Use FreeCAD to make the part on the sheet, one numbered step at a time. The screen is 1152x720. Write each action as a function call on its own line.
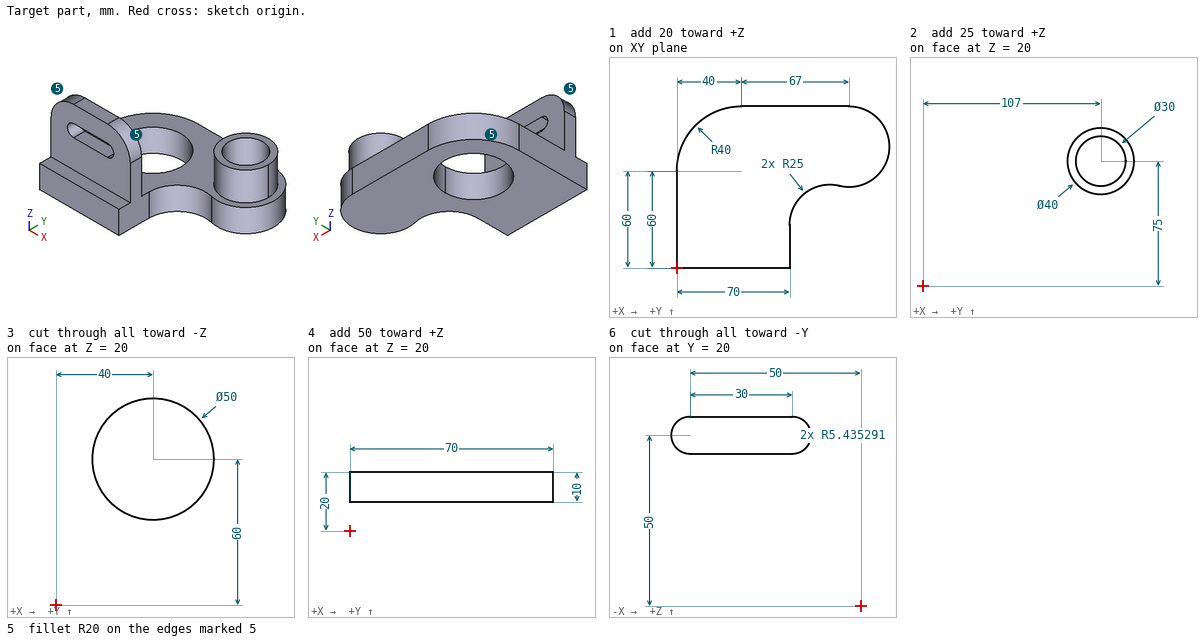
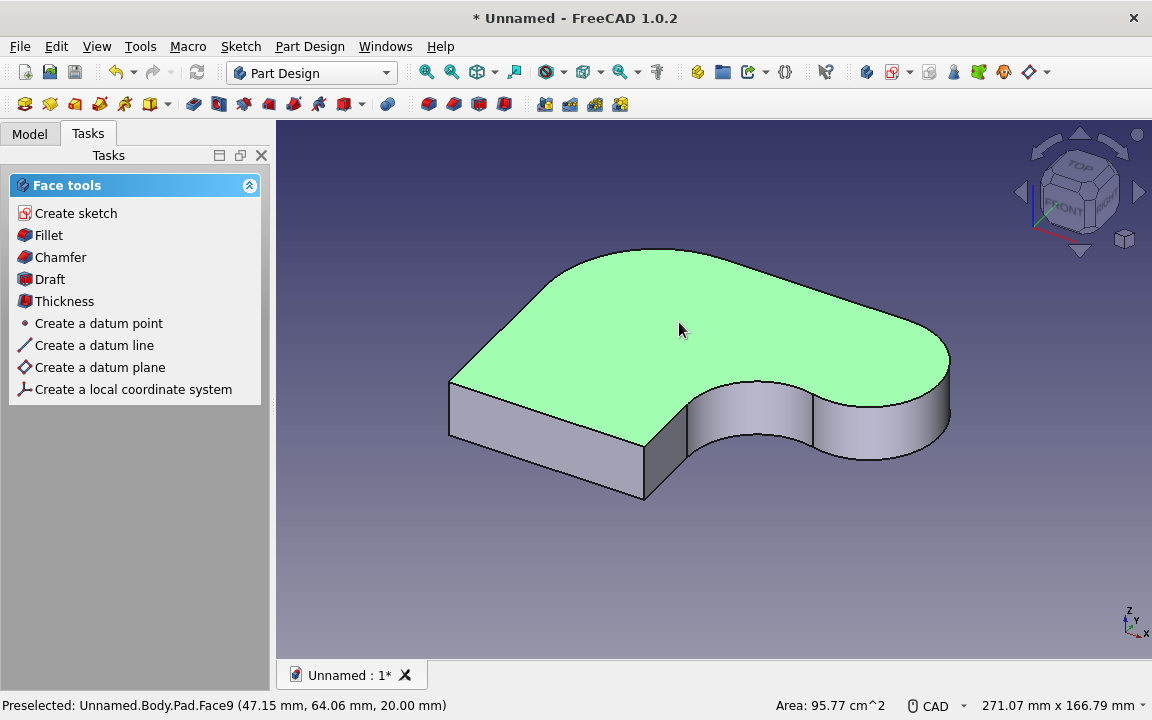
click(892, 72)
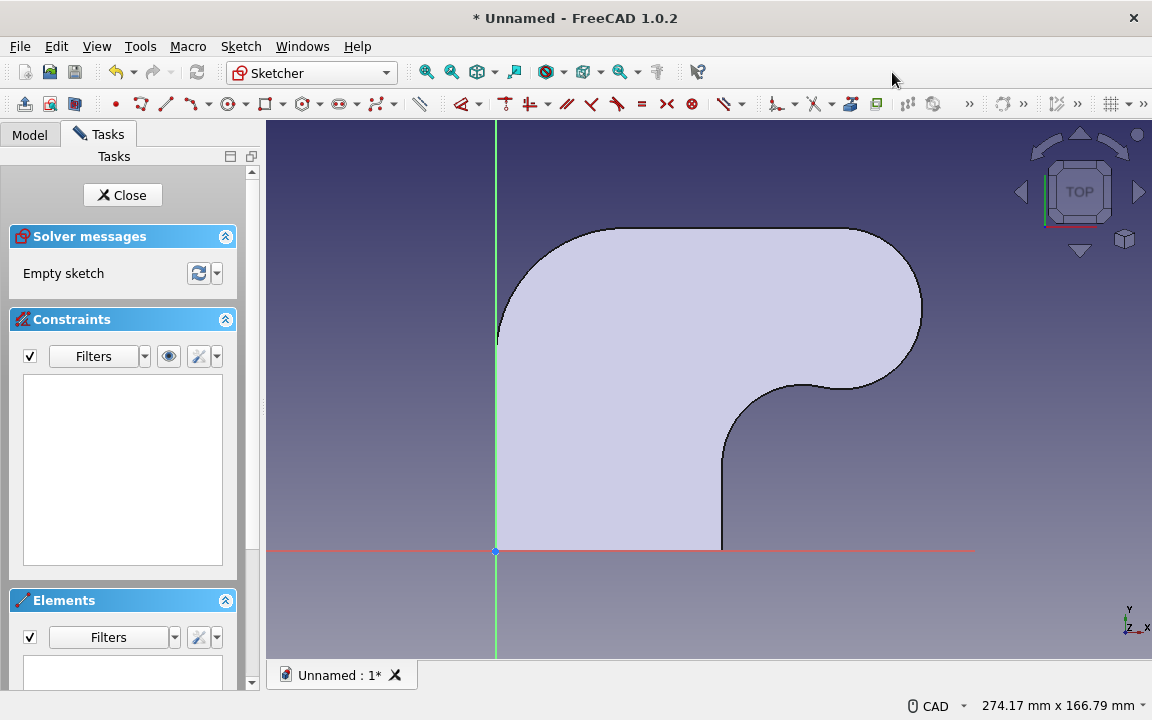
scroll(959, 262, up, 5)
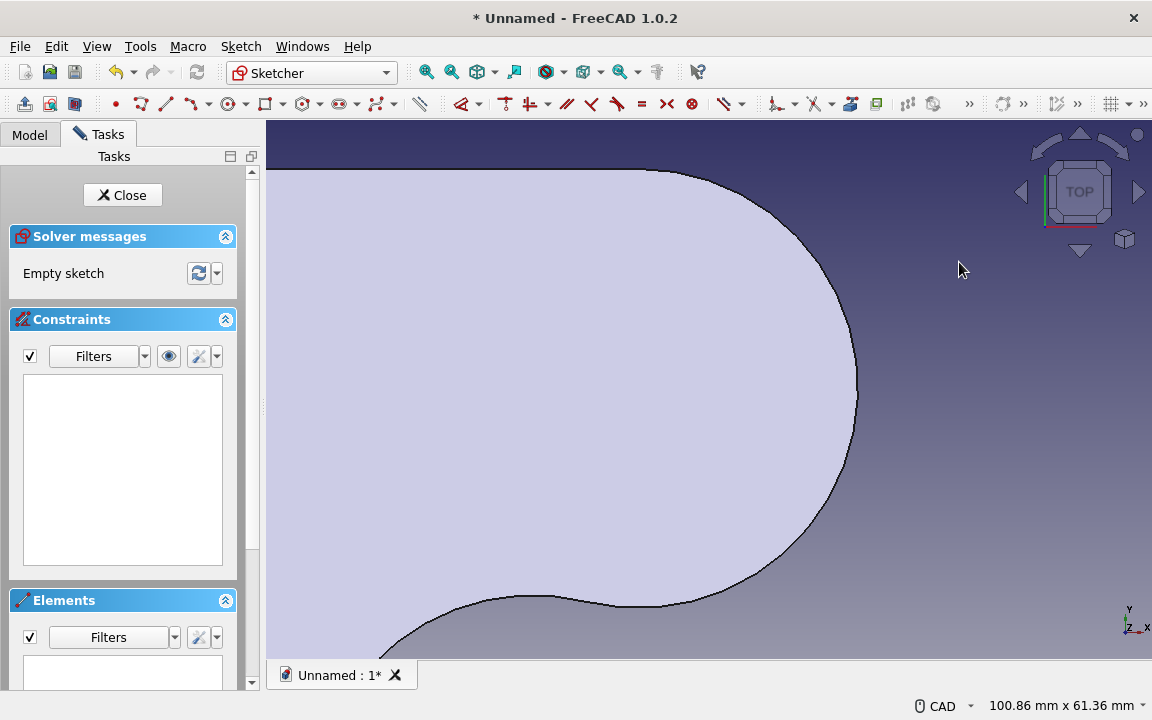
click(228, 104)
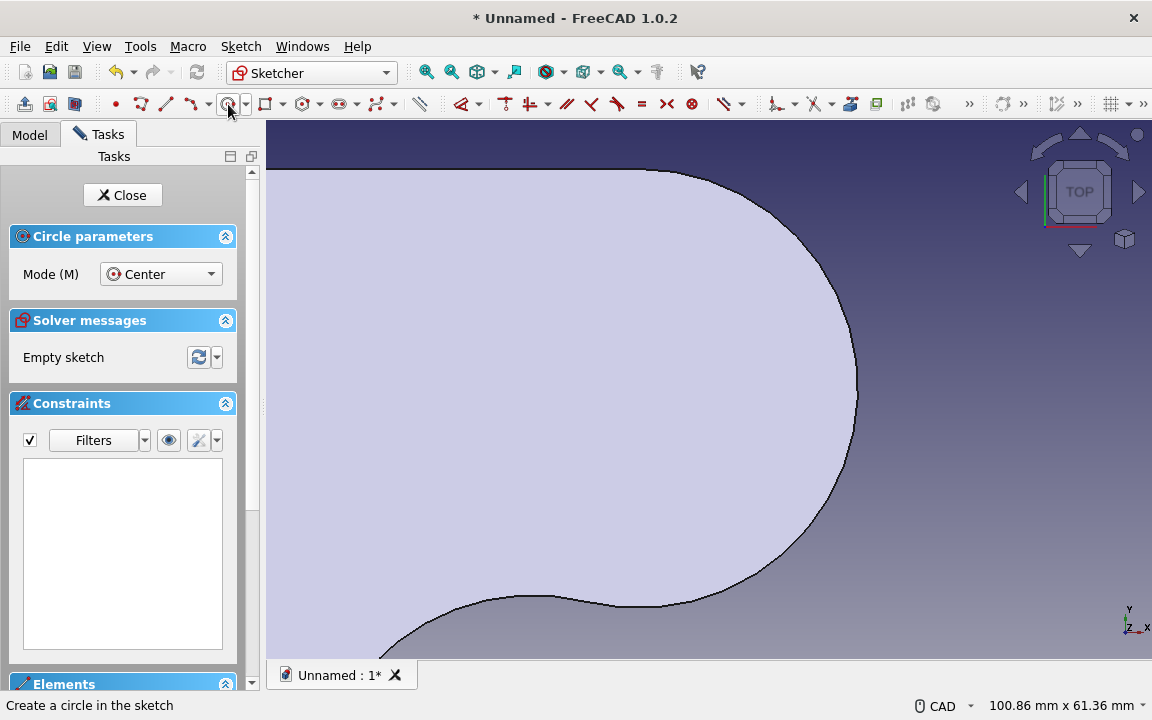
click(638, 389)
move(763, 264)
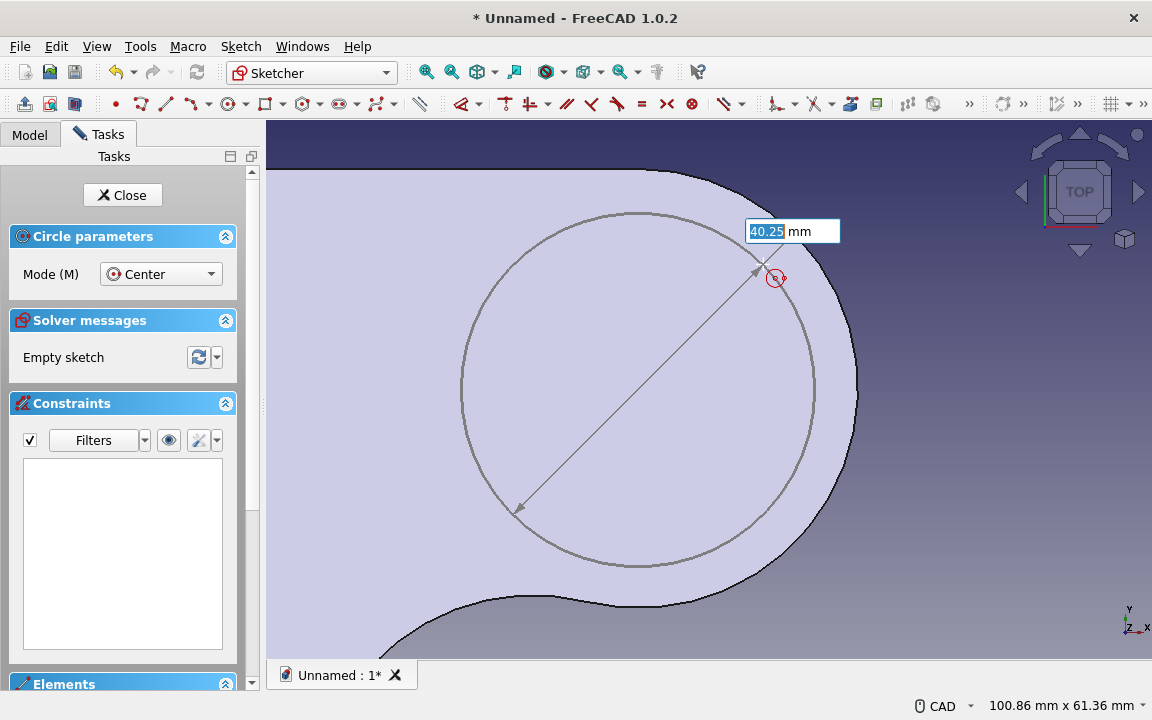
text(40)
key(Return)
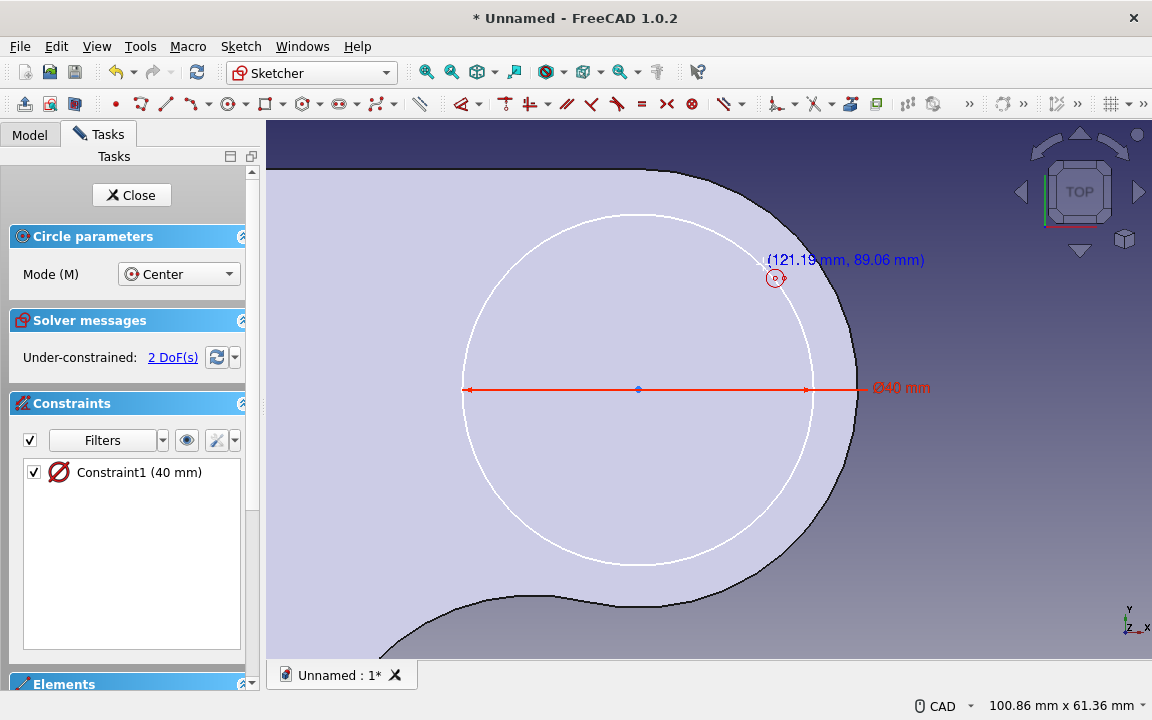
click(638, 390)
move(732, 295)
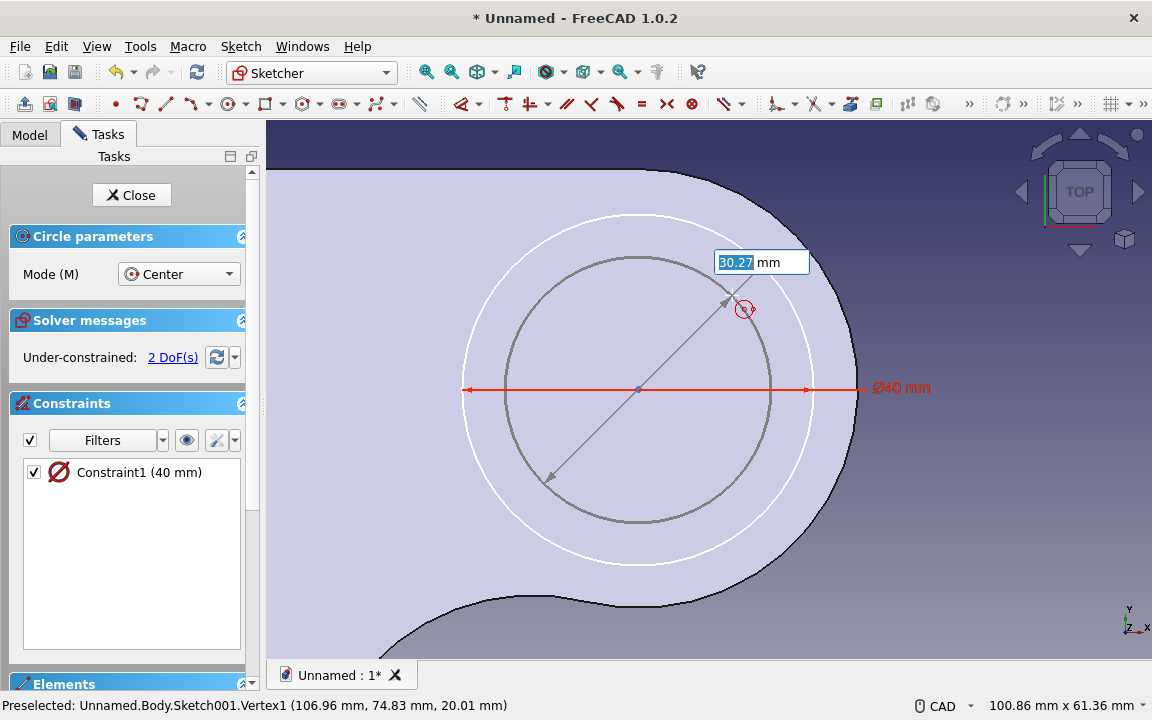
text(30)
key(Return)
key(Escape)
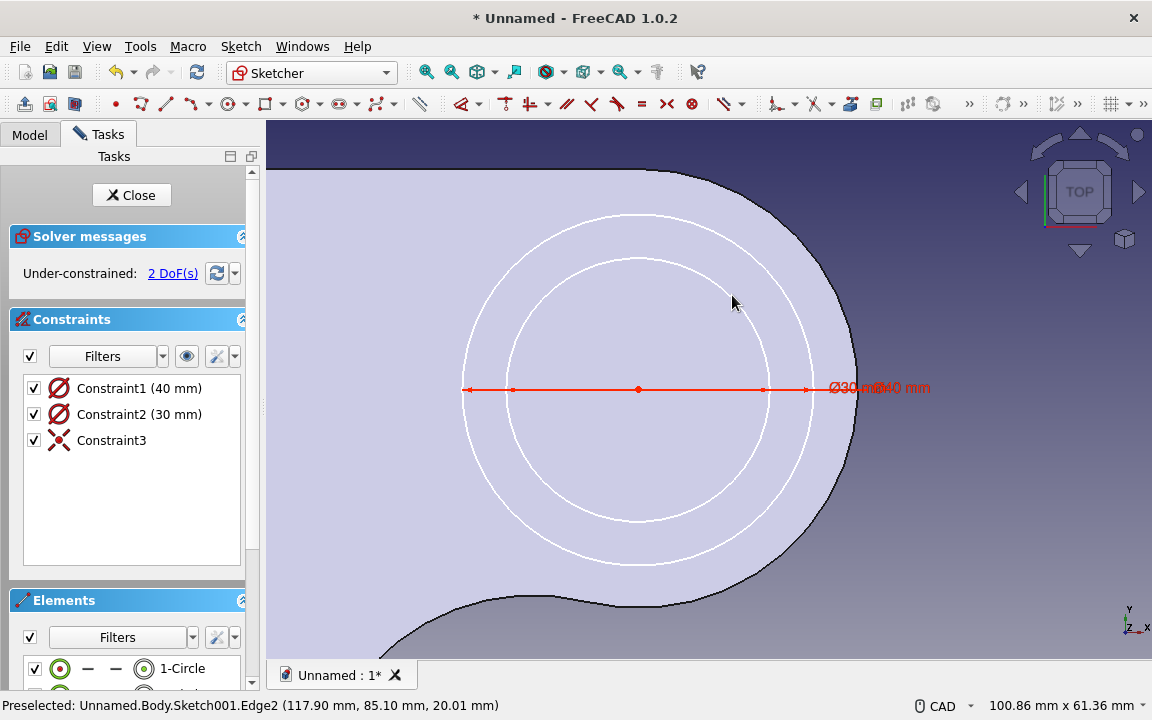
click(460, 104)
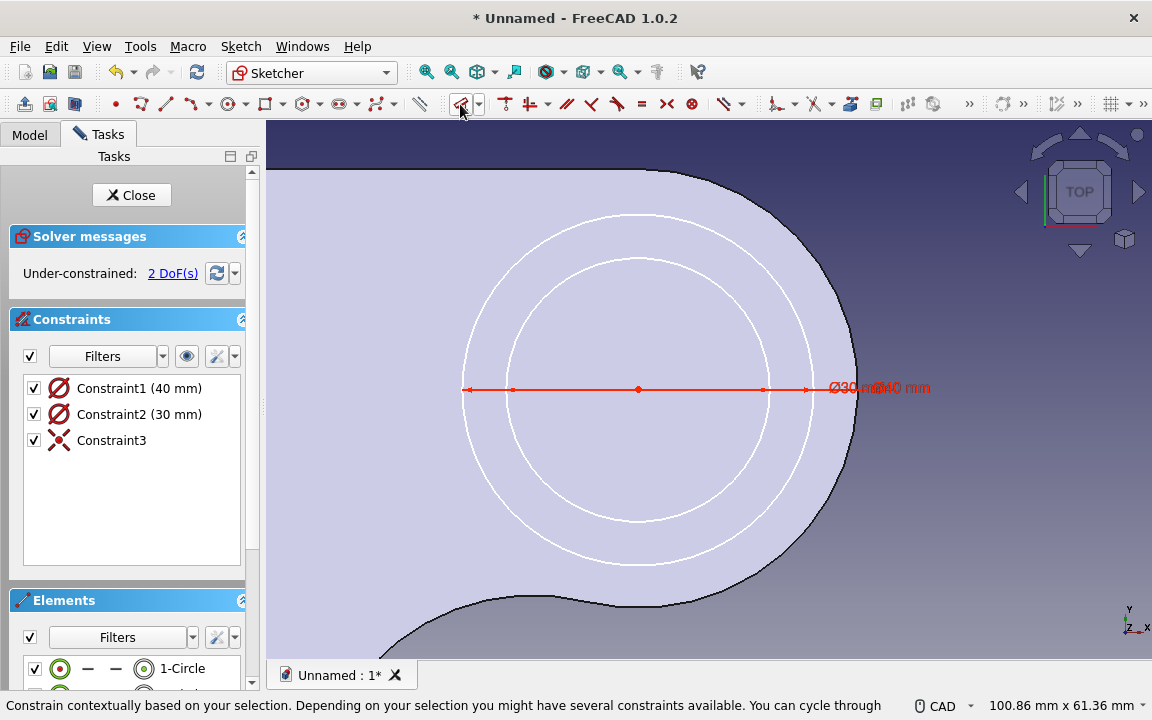
click(638, 390)
click(672, 455)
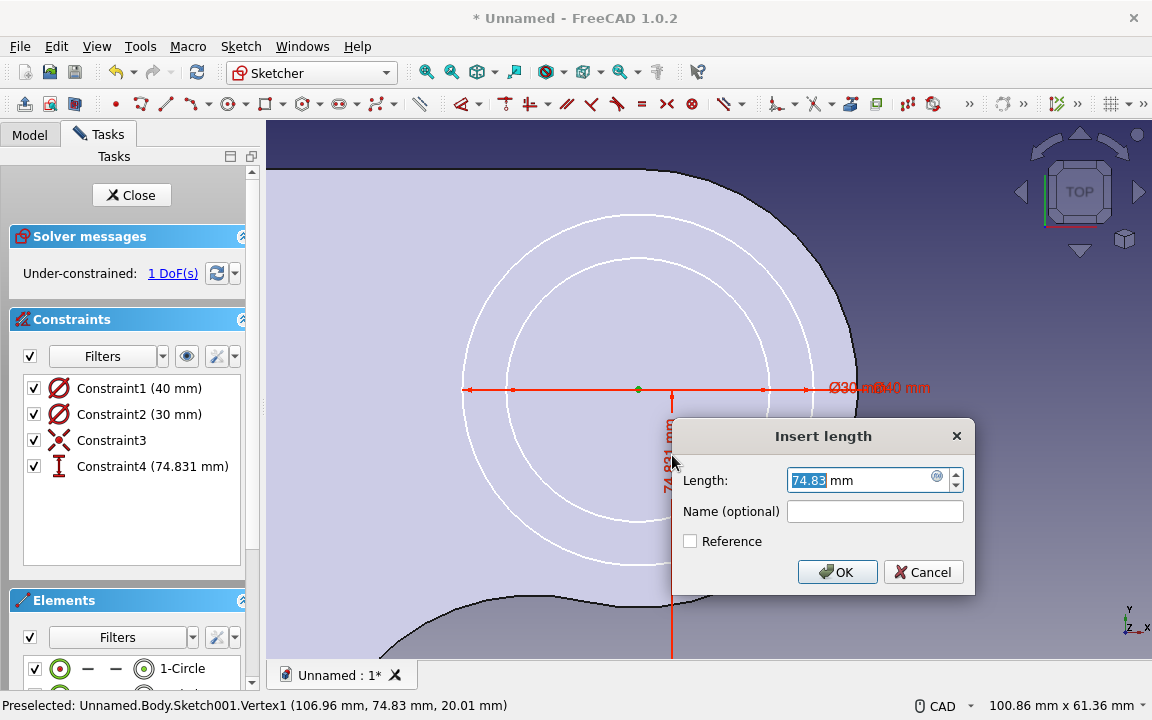
text(75)
key(Return)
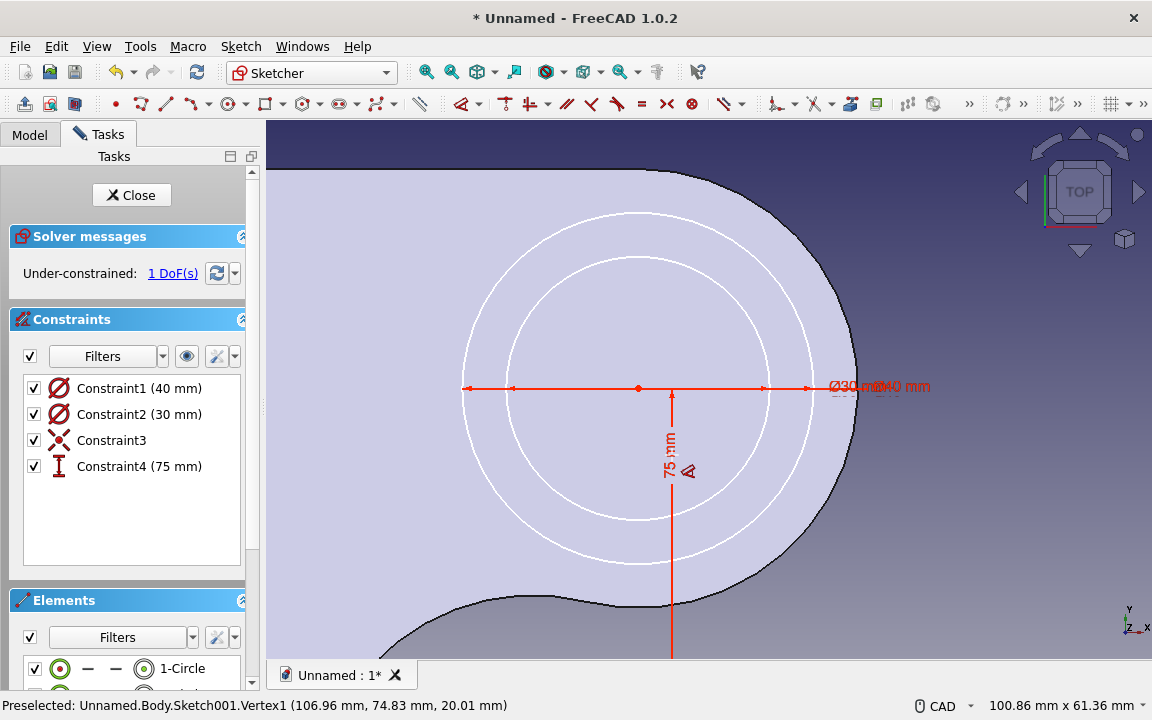
click(638, 389)
click(387, 355)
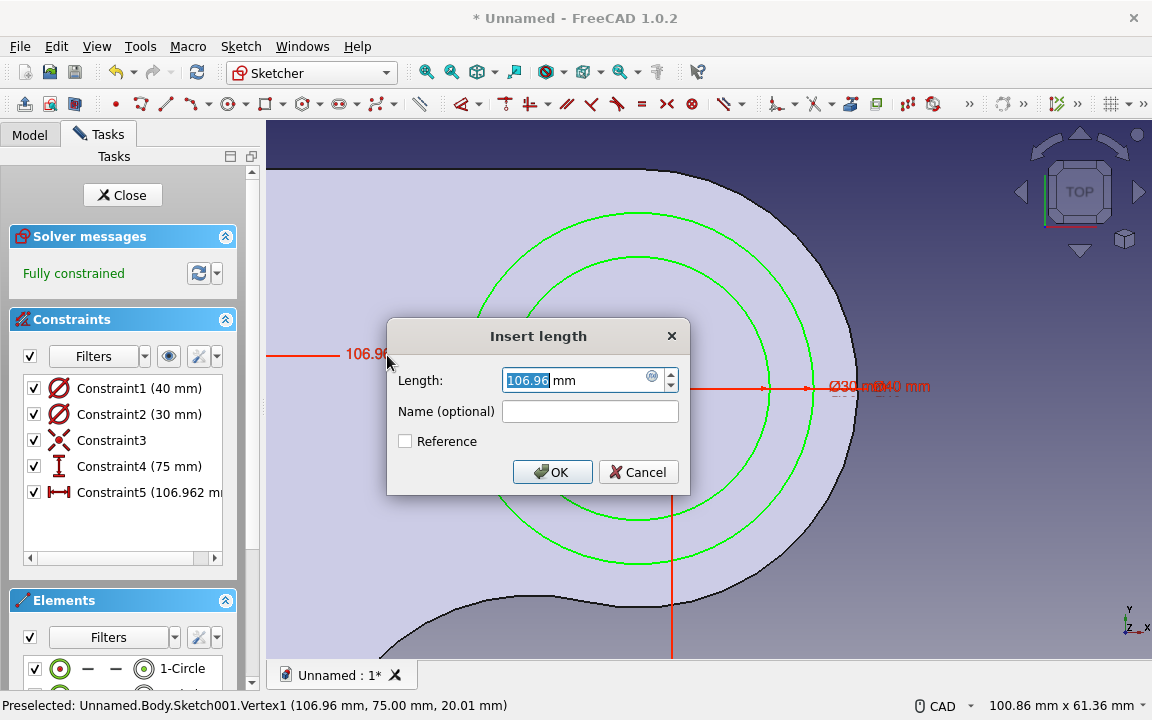
text(107)
key(Return)
key(Escape)